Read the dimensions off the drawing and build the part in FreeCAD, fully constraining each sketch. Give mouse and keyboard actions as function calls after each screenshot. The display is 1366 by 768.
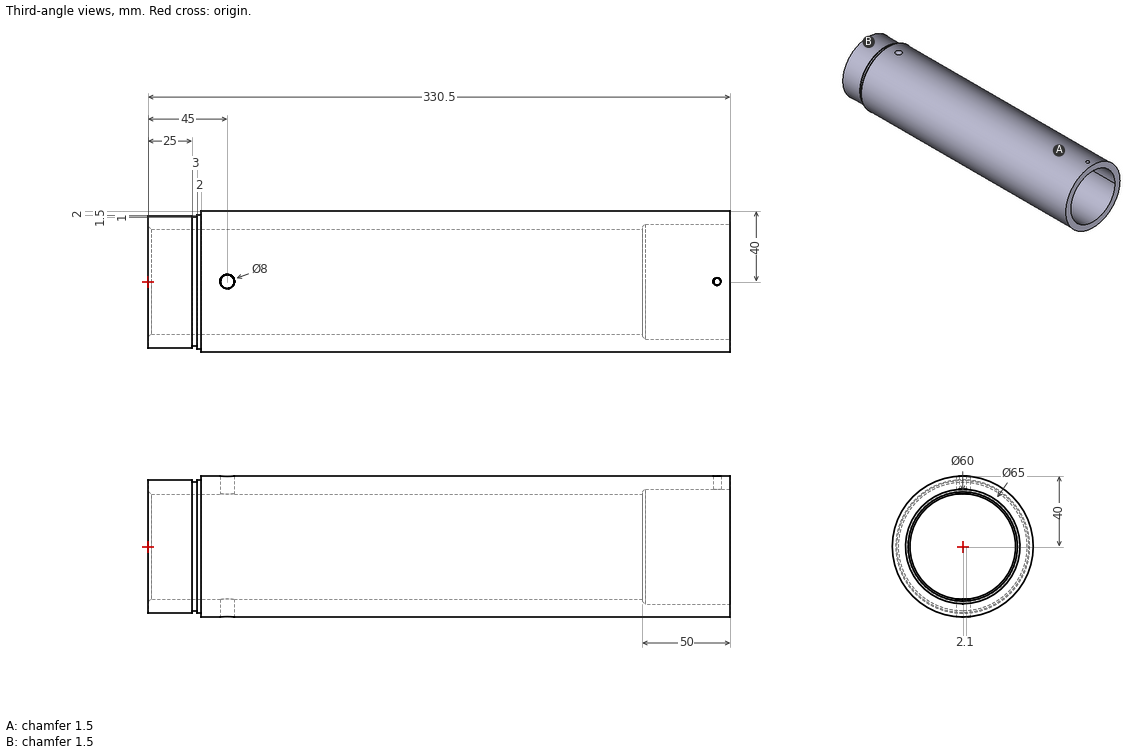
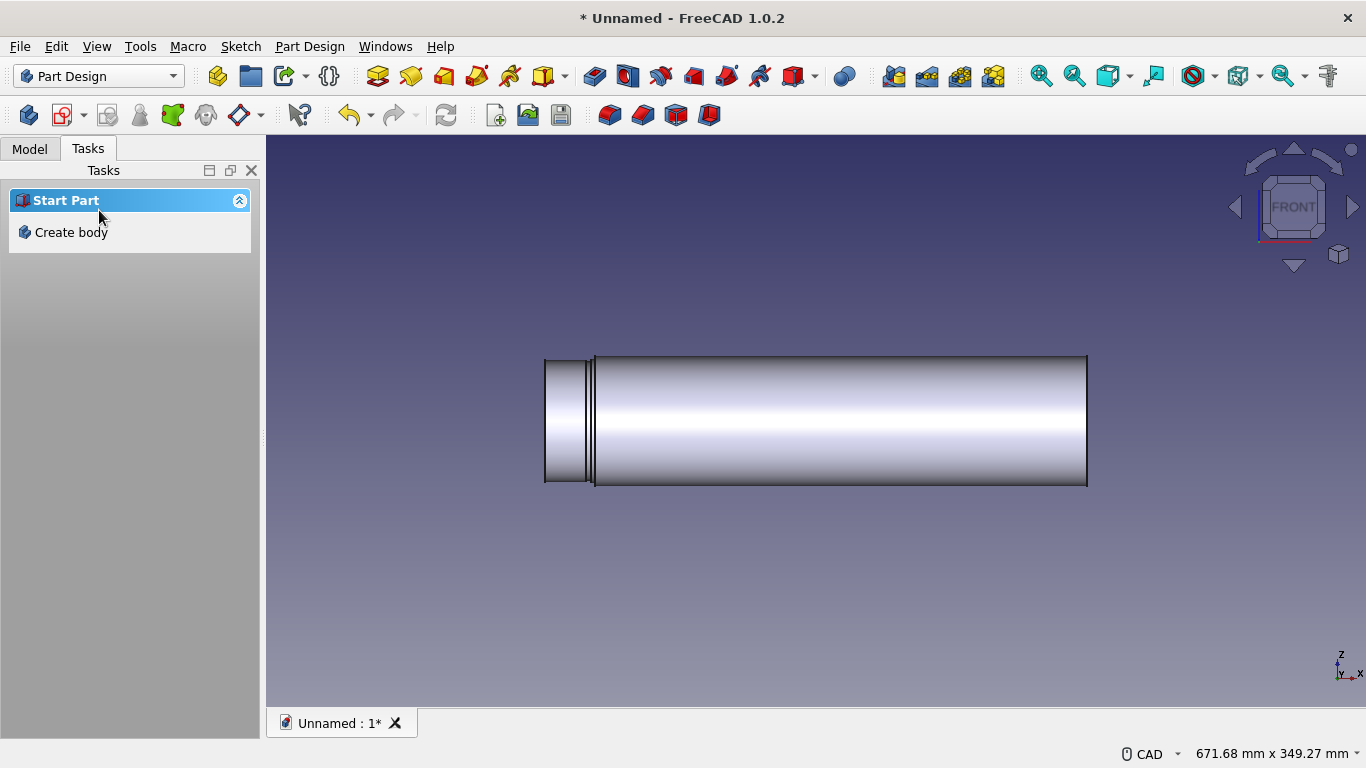
key(3)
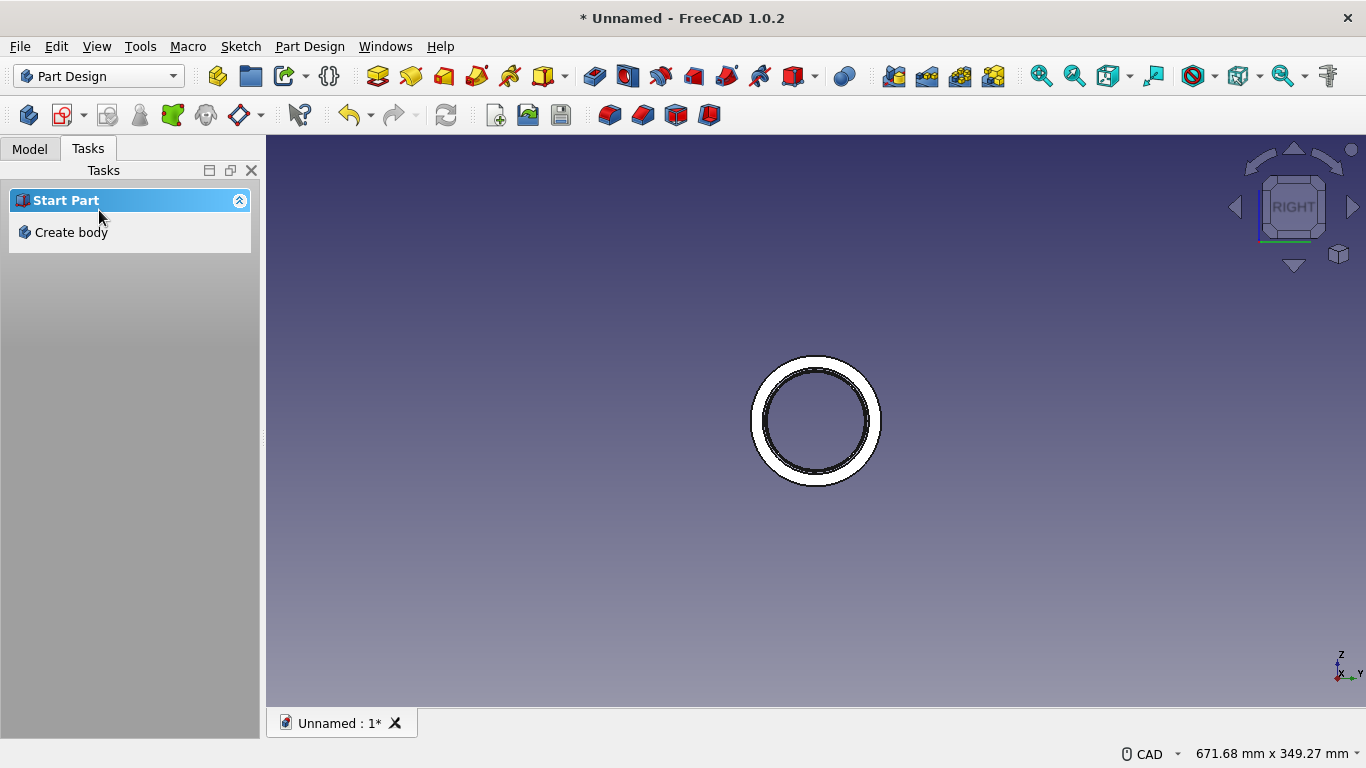
click(1042, 76)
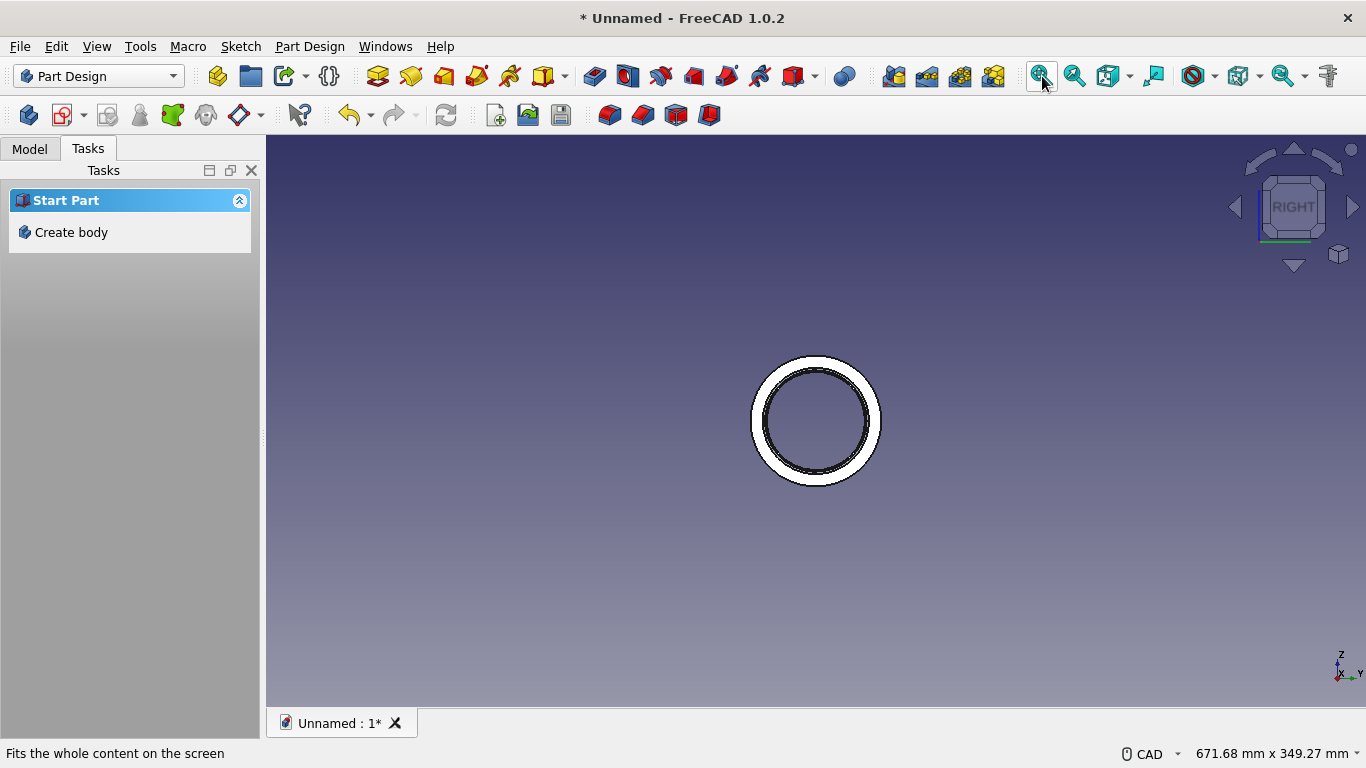
key(5)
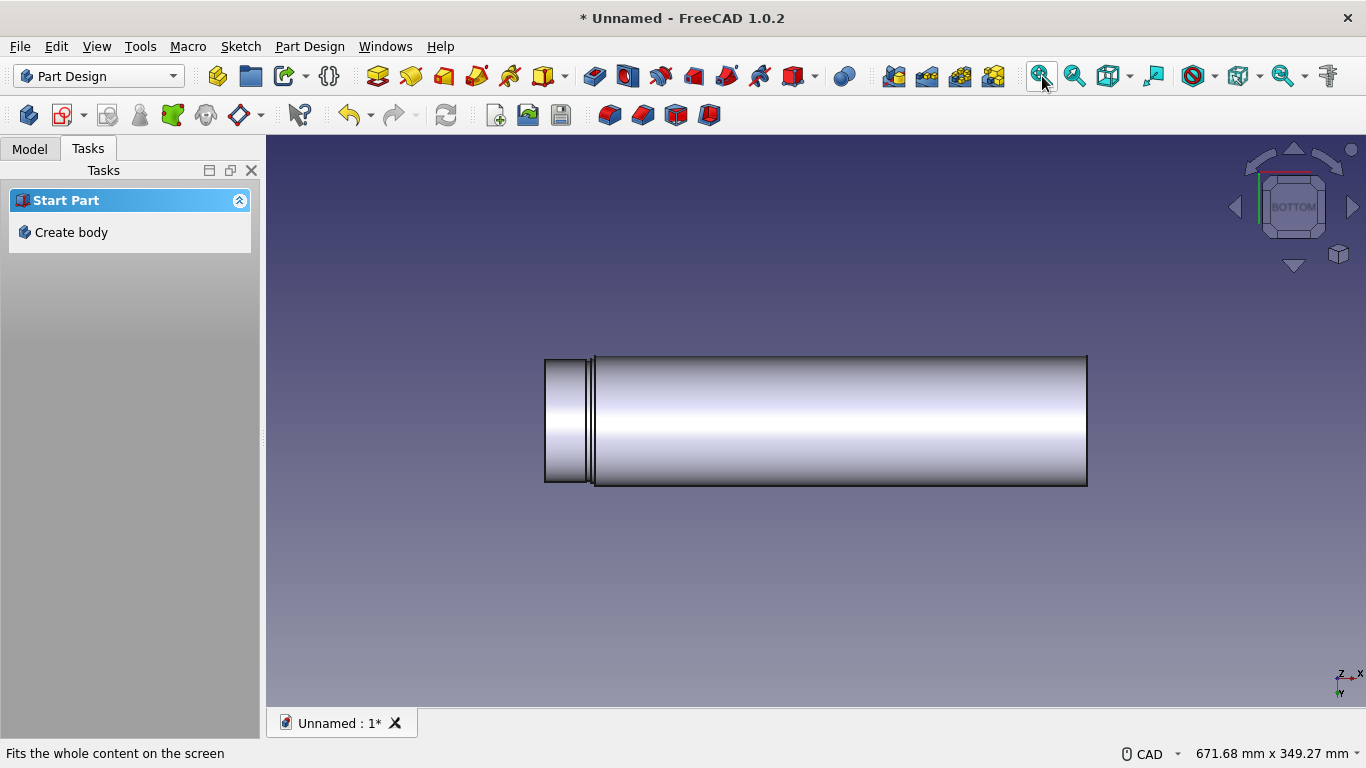
key(4)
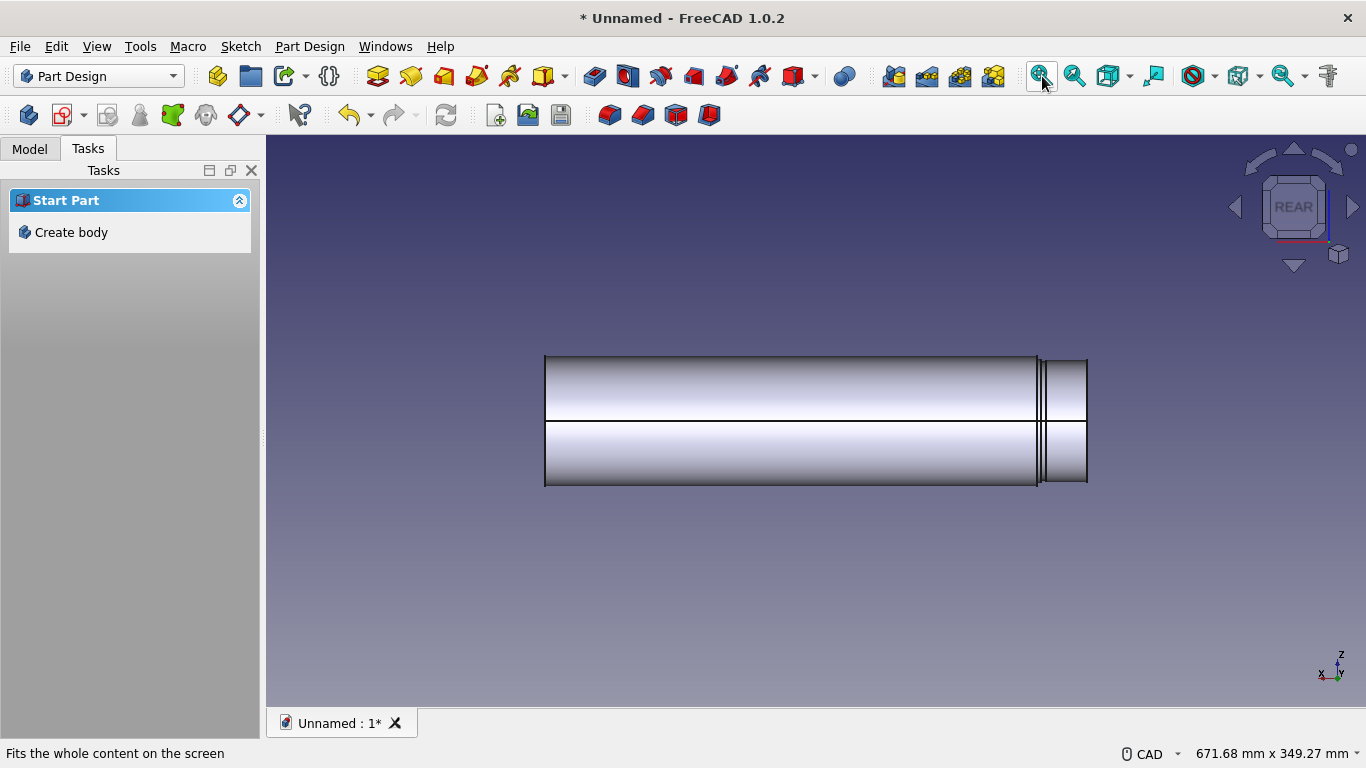
key(6)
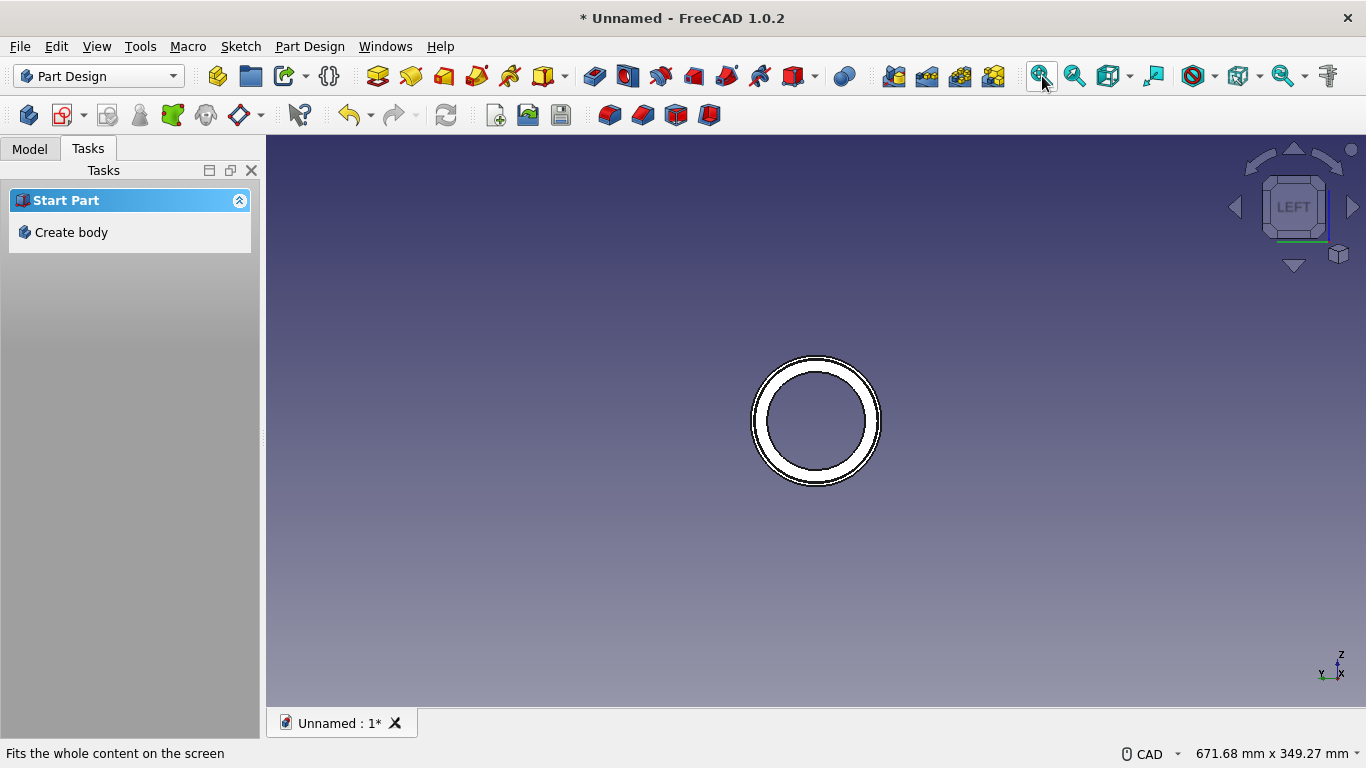
click(1042, 76)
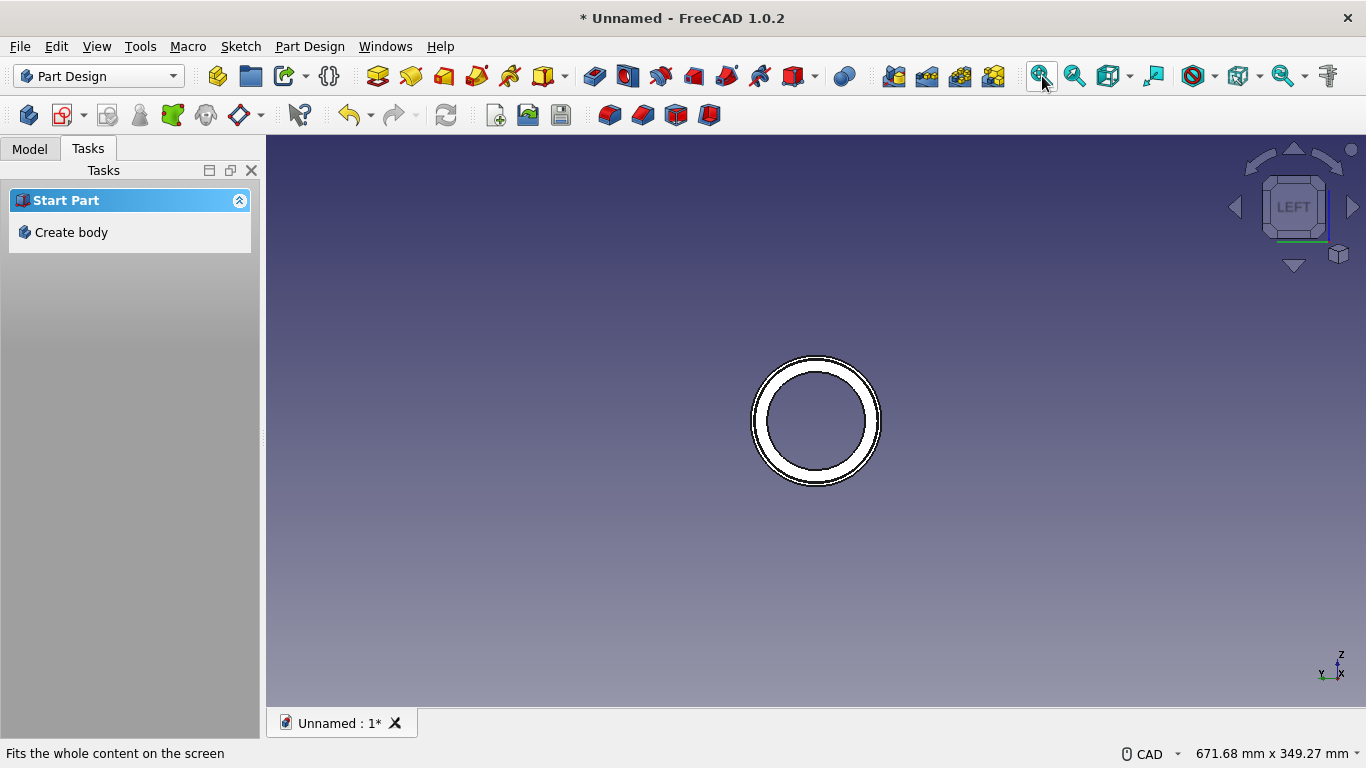
click(865, 420)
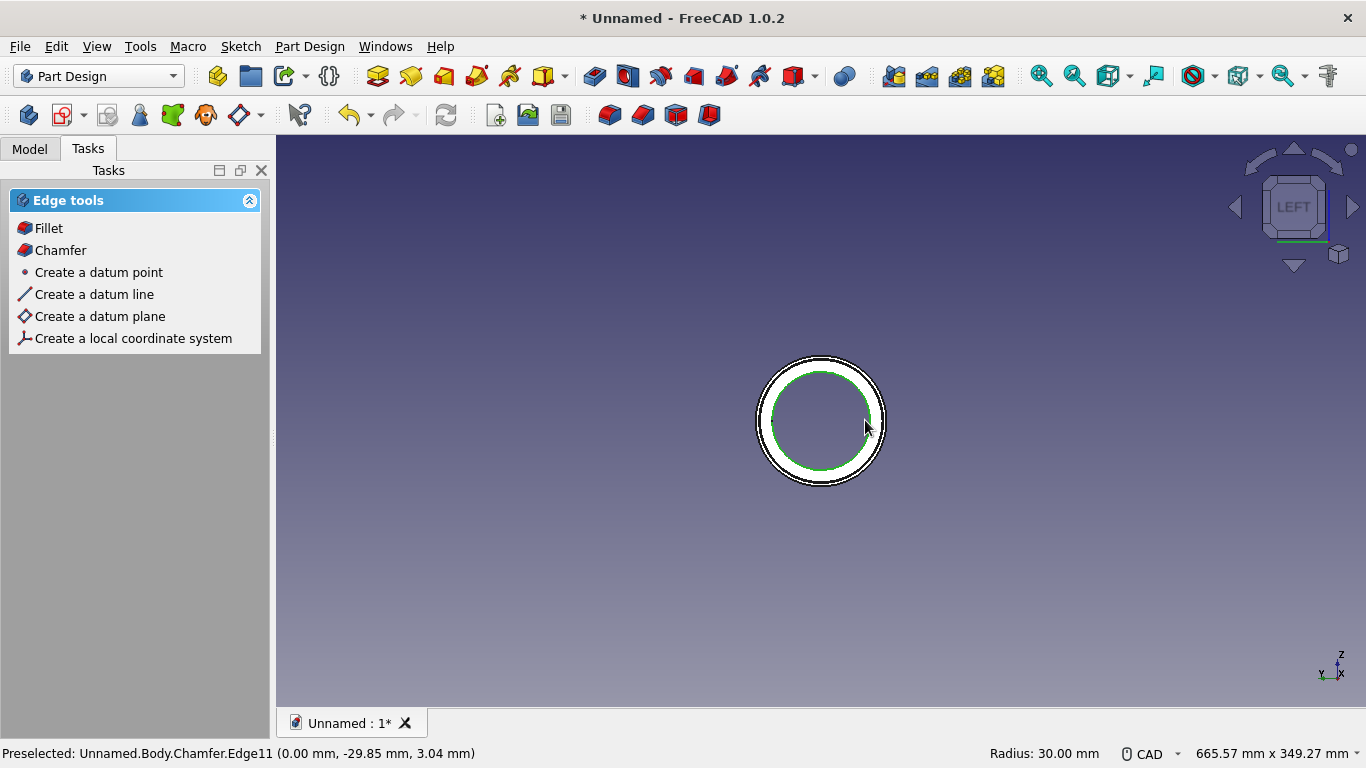
click(643, 116)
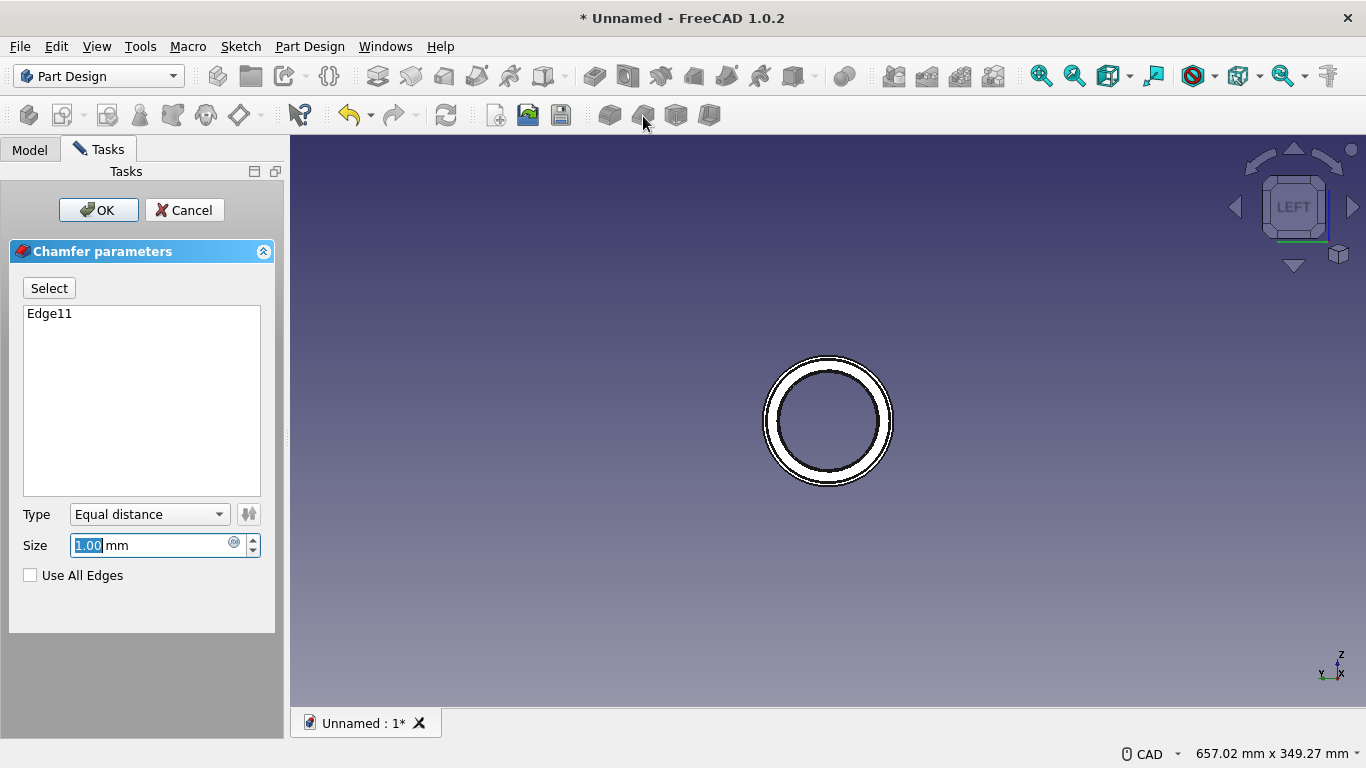
text(1.5)
key(Tab)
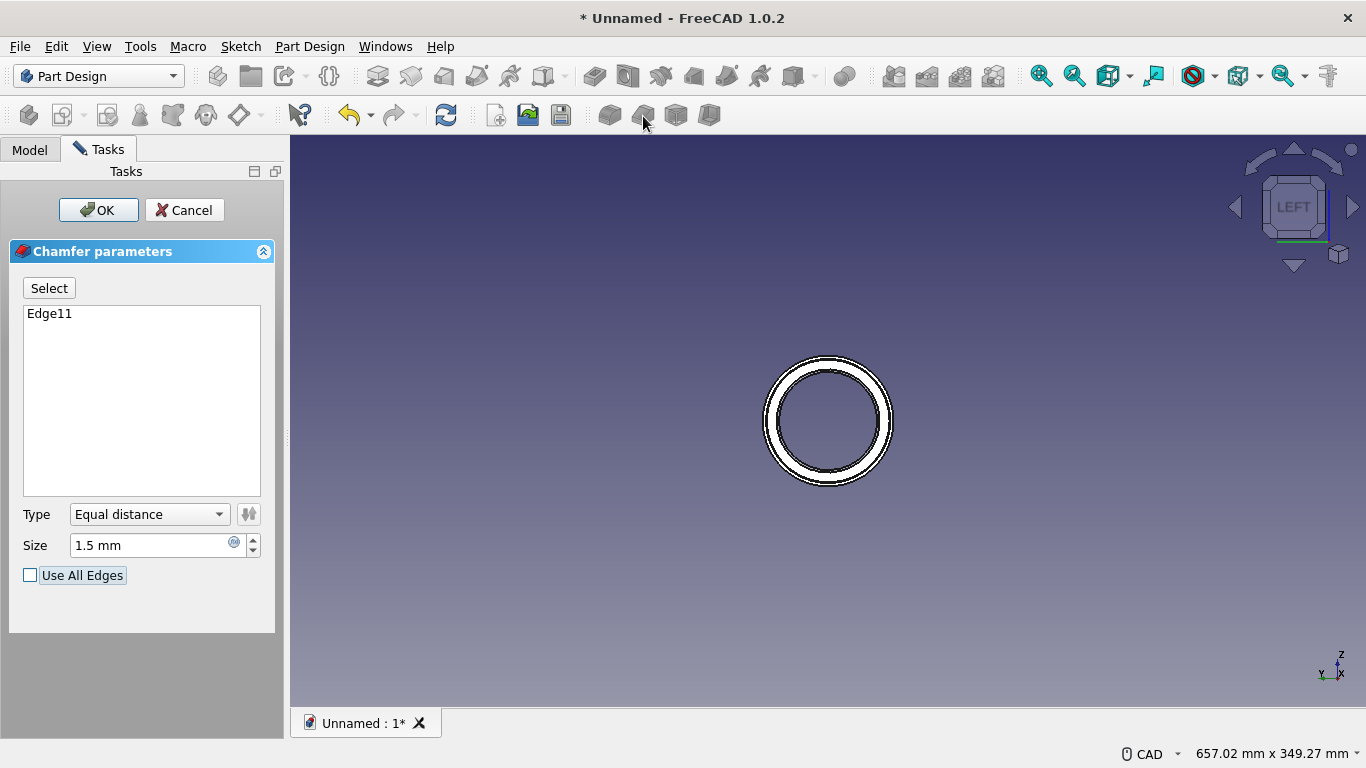
click(99, 210)